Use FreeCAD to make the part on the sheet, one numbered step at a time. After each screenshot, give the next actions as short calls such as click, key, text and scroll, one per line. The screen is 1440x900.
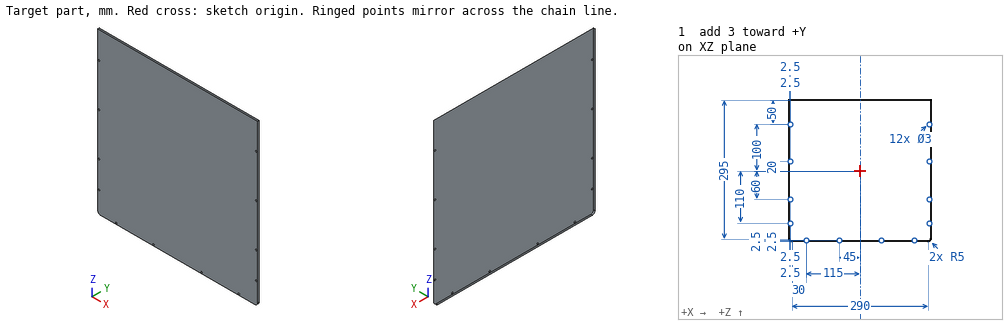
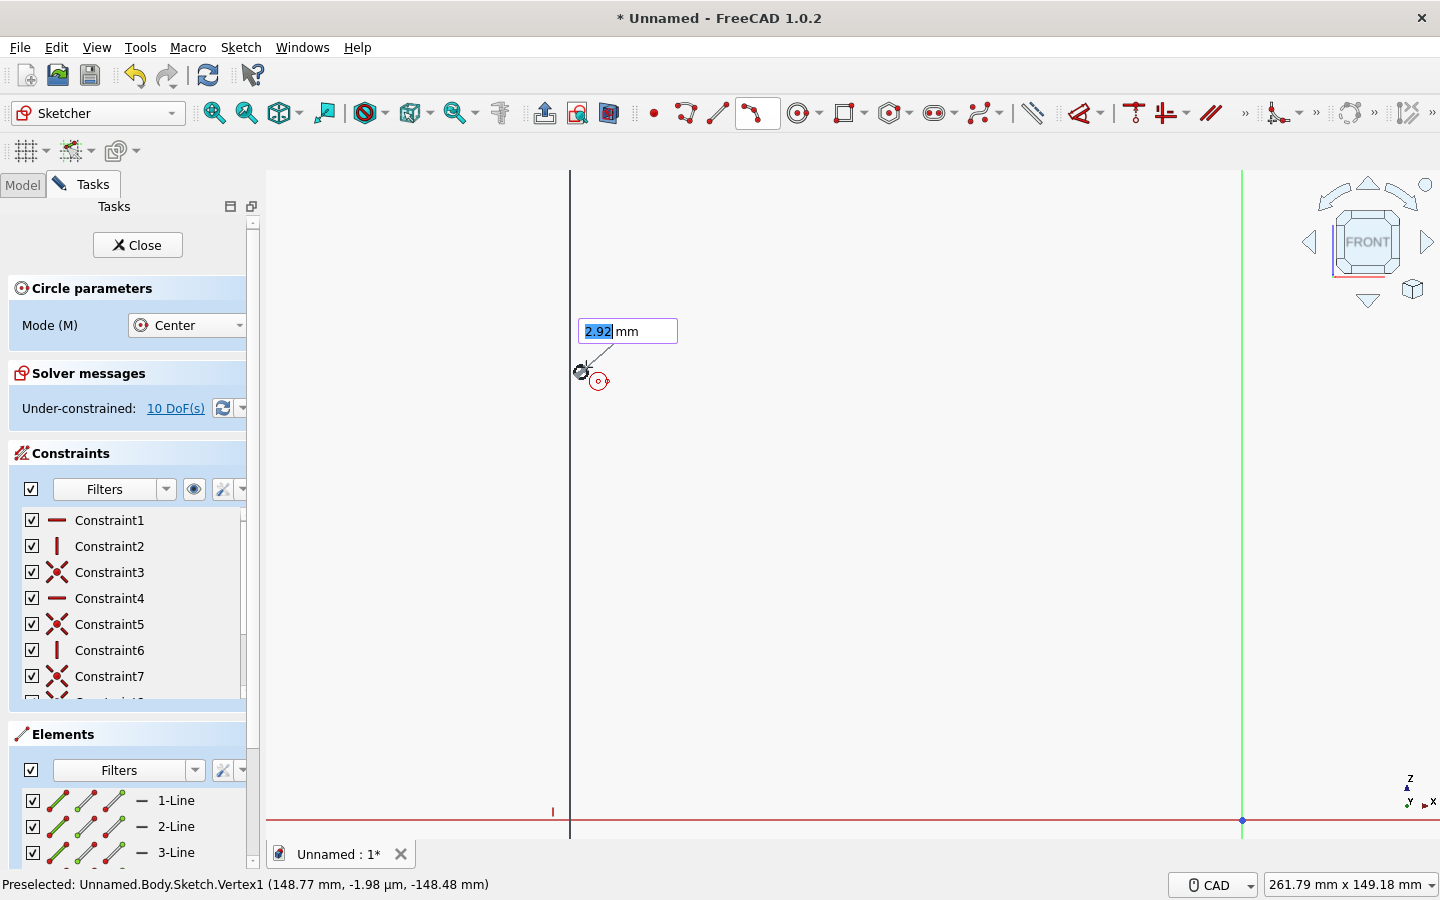
text(3)
key(Return)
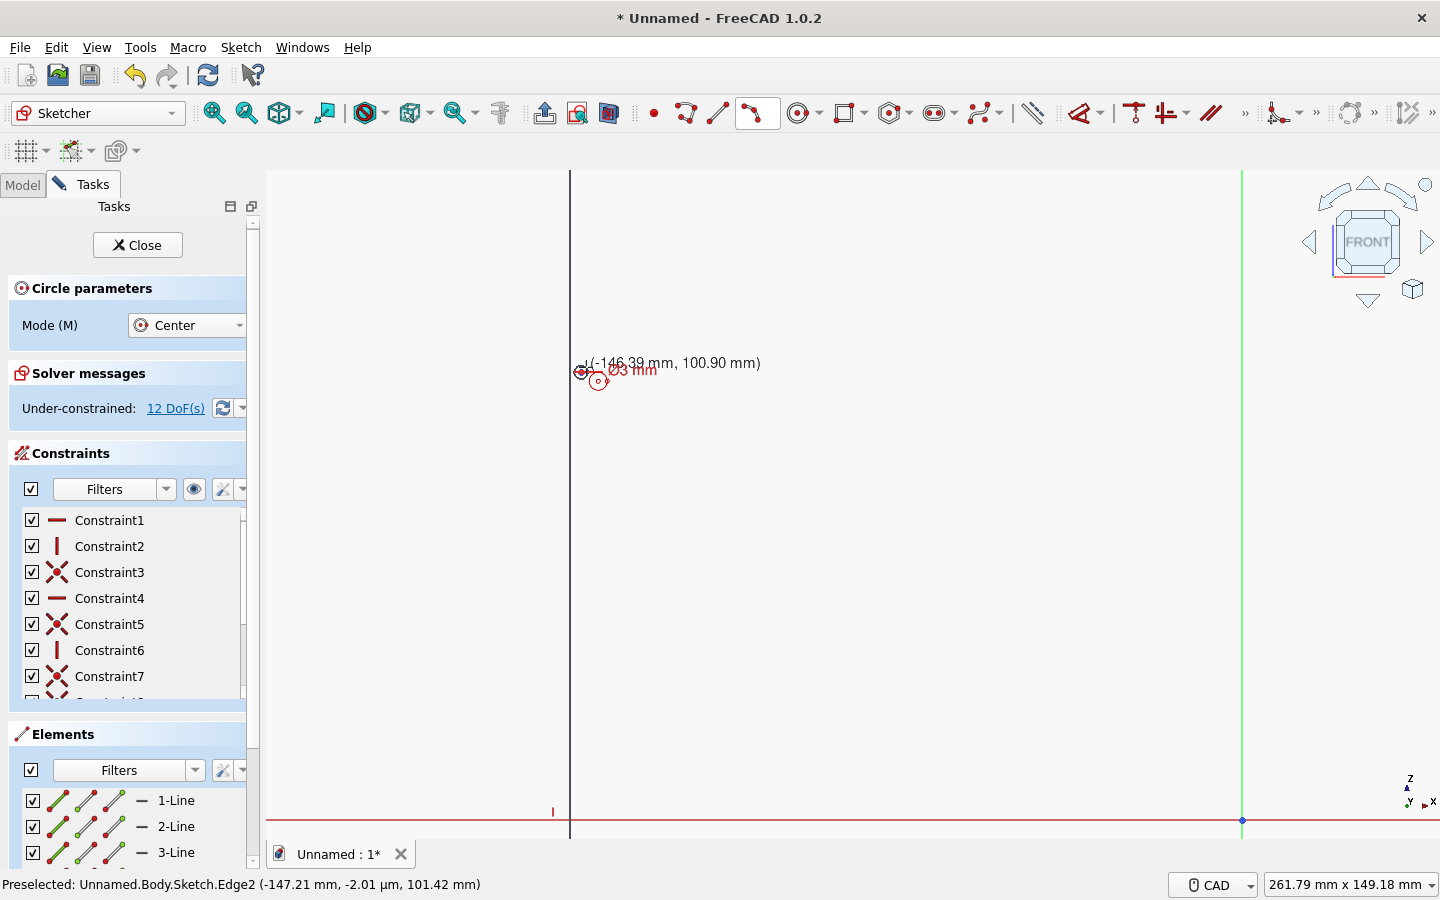
scroll(581, 731, up, 7)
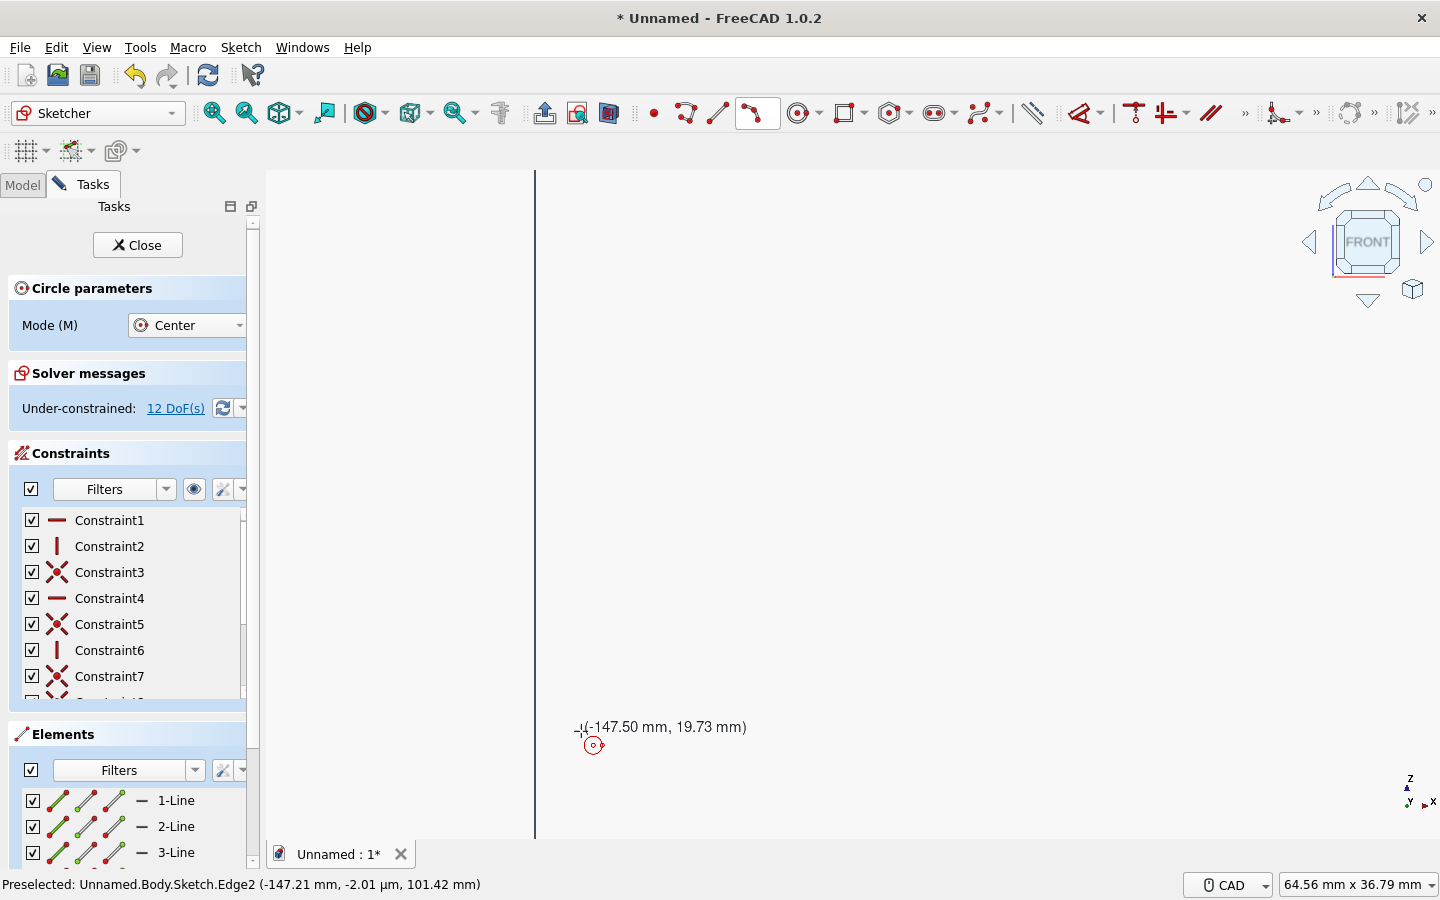
click(580, 728)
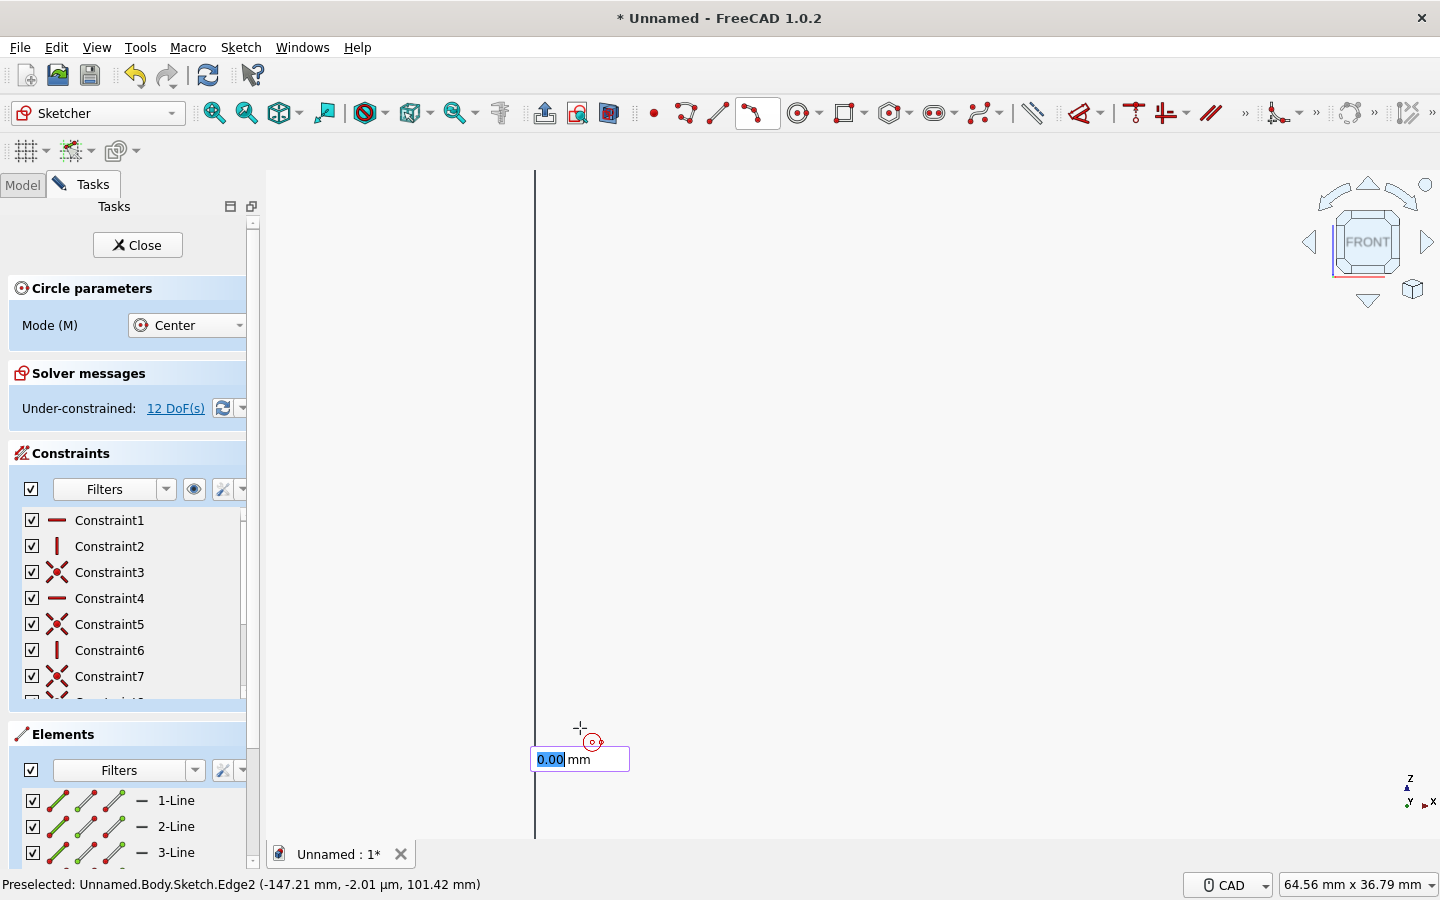
scroll(586, 457, down, 13)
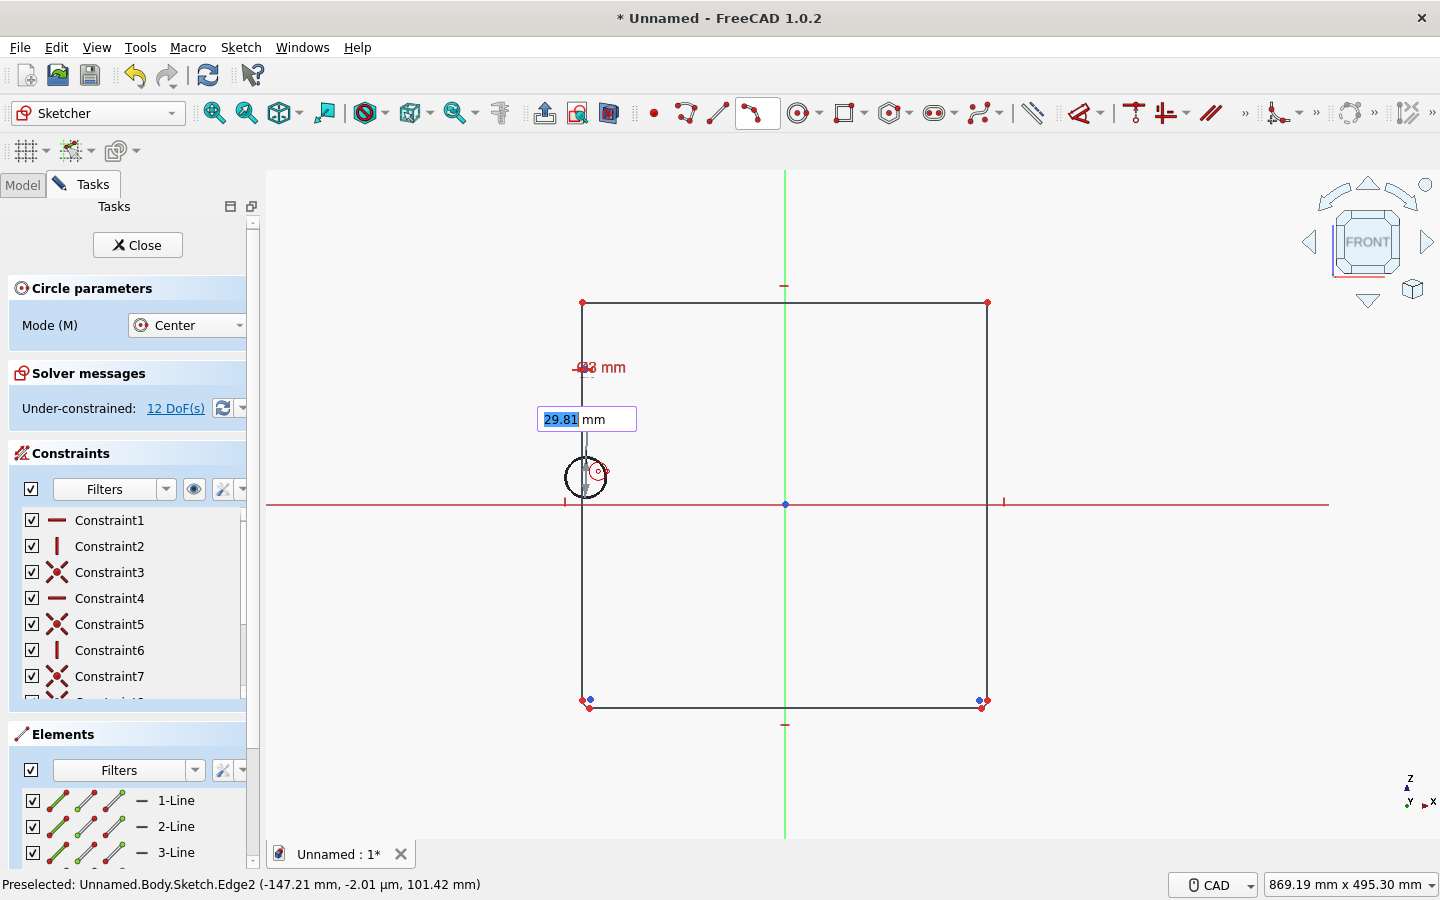
scroll(587, 476, up, 6)
move(587, 475)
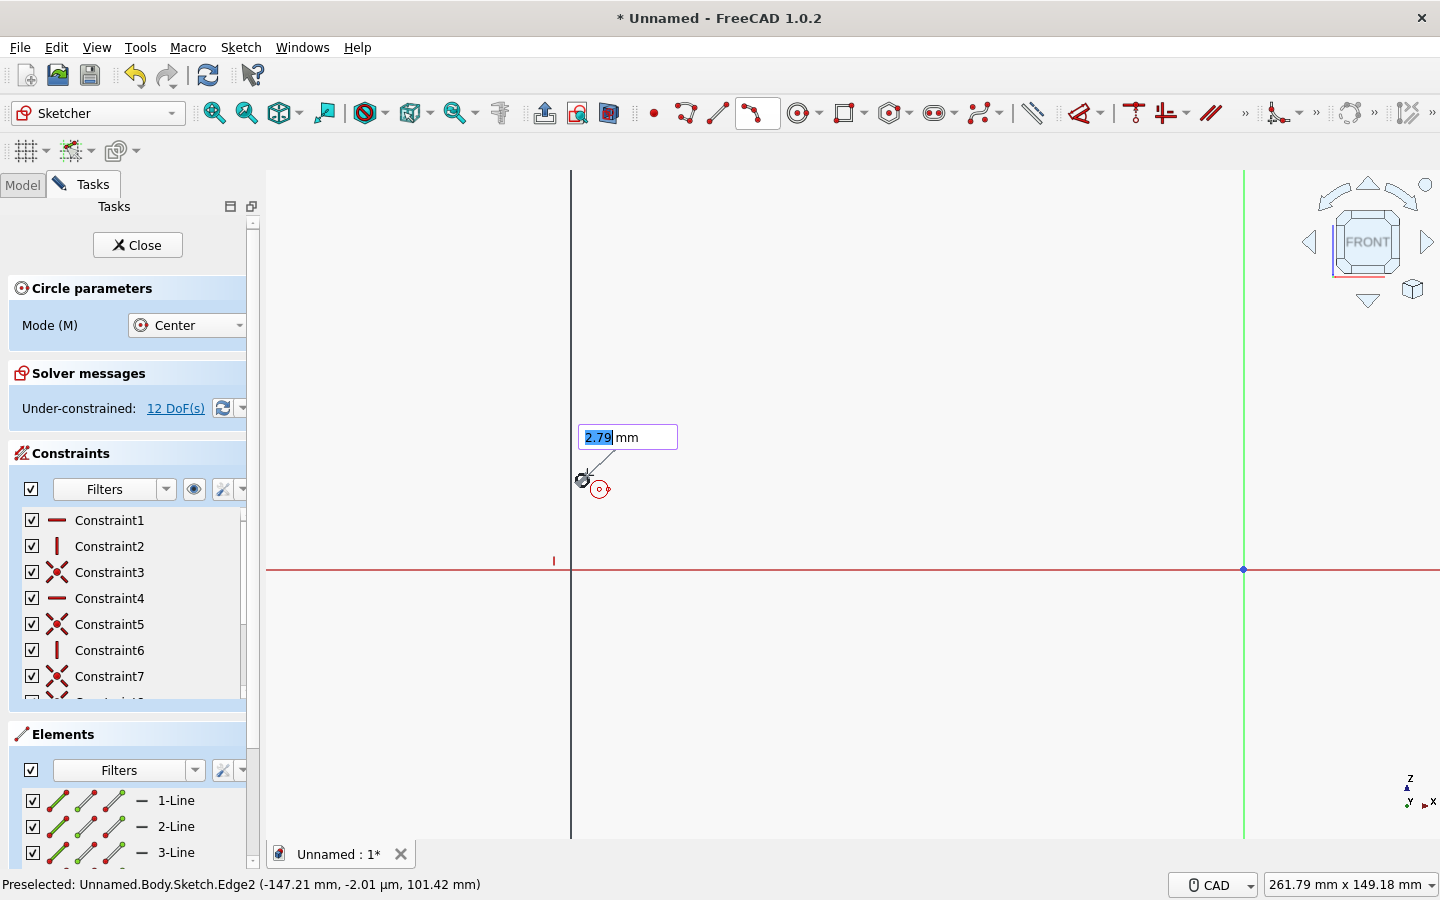
text(3)
key(Return)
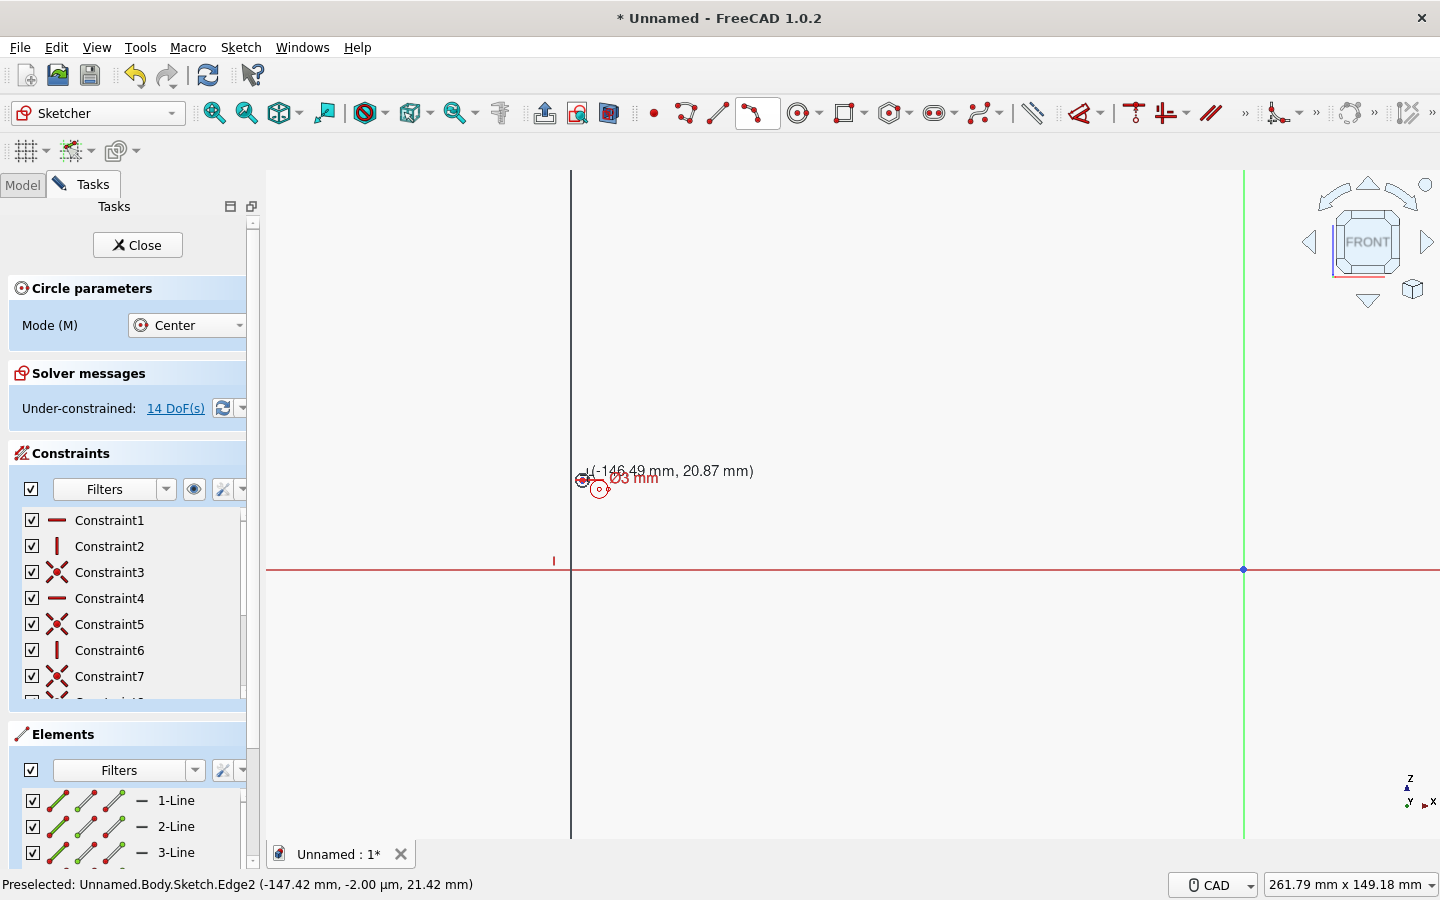
scroll(586, 476, down, 6)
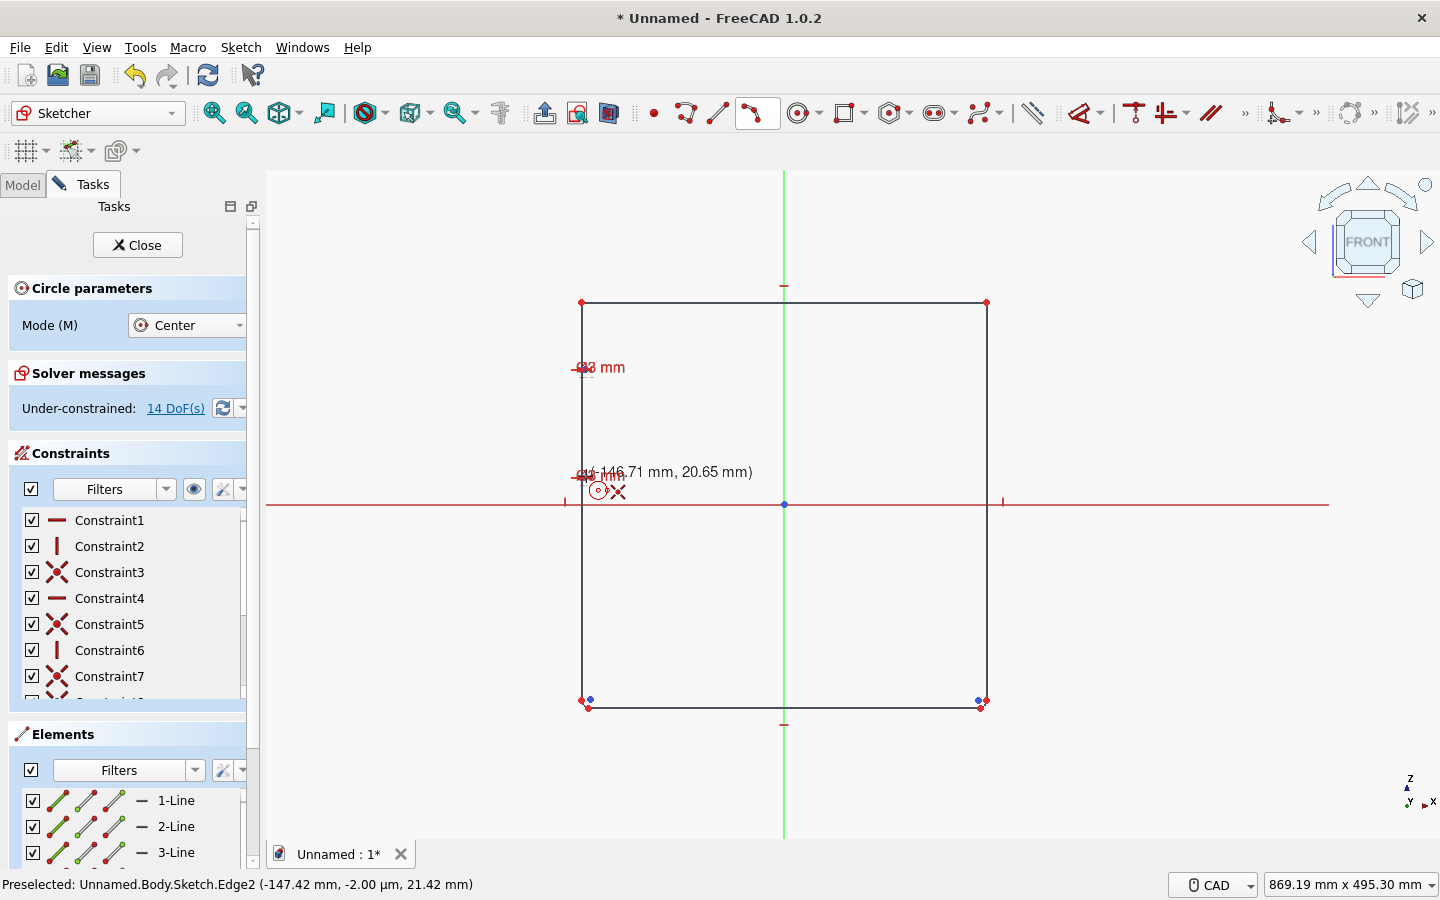
scroll(984, 369, up, 13)